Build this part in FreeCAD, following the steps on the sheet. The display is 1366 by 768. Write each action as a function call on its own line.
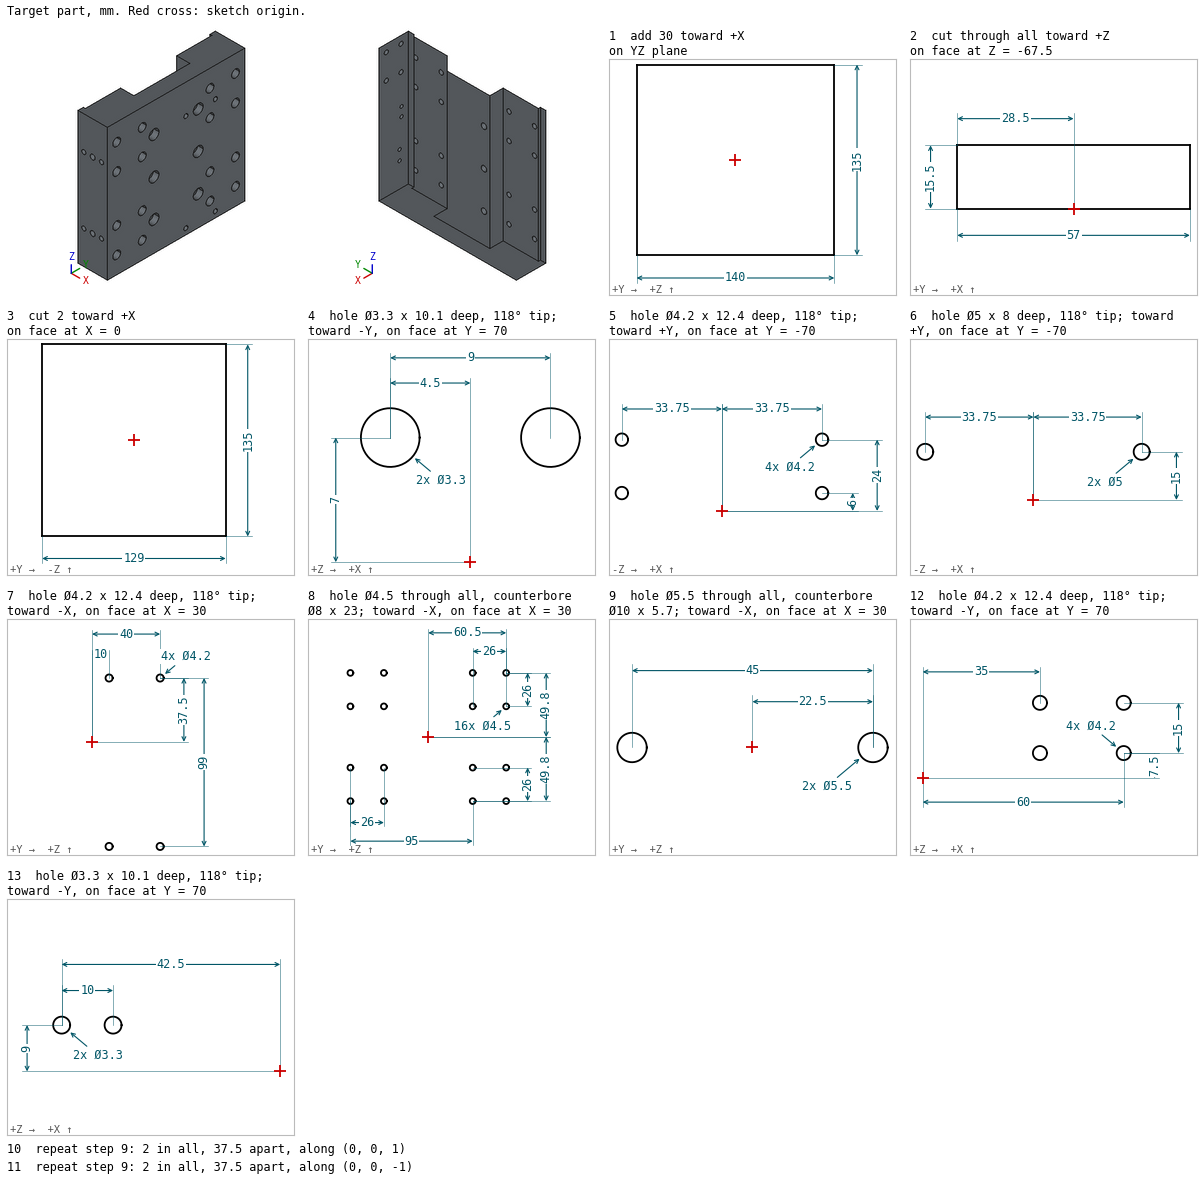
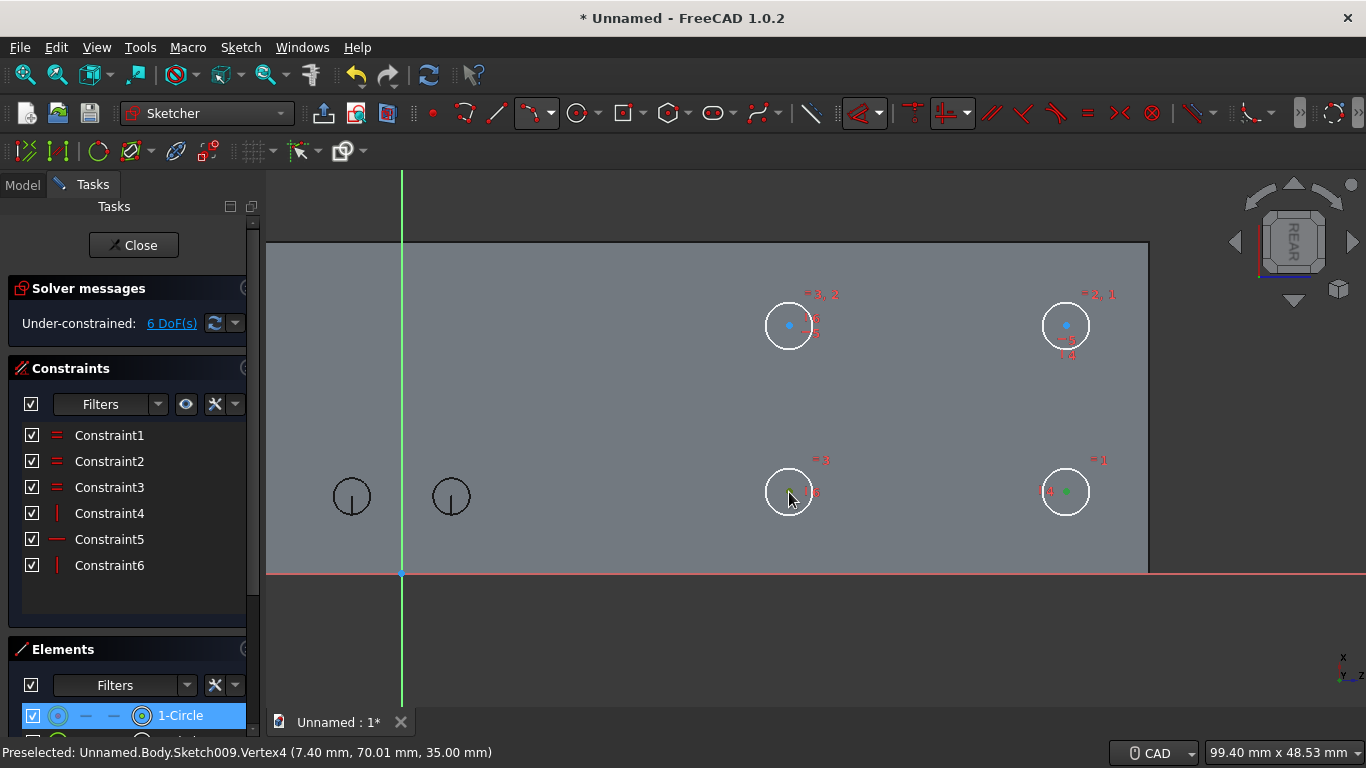
click(970, 114)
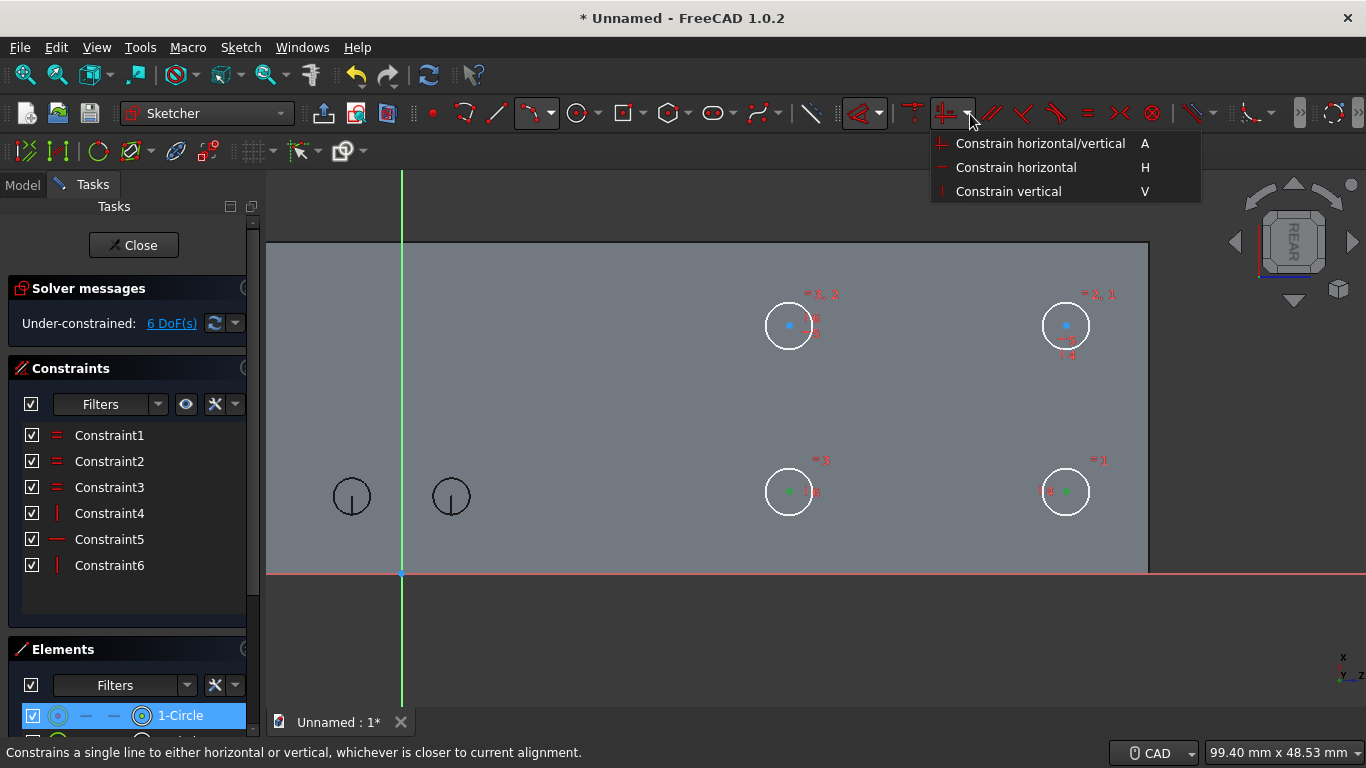
click(1066, 167)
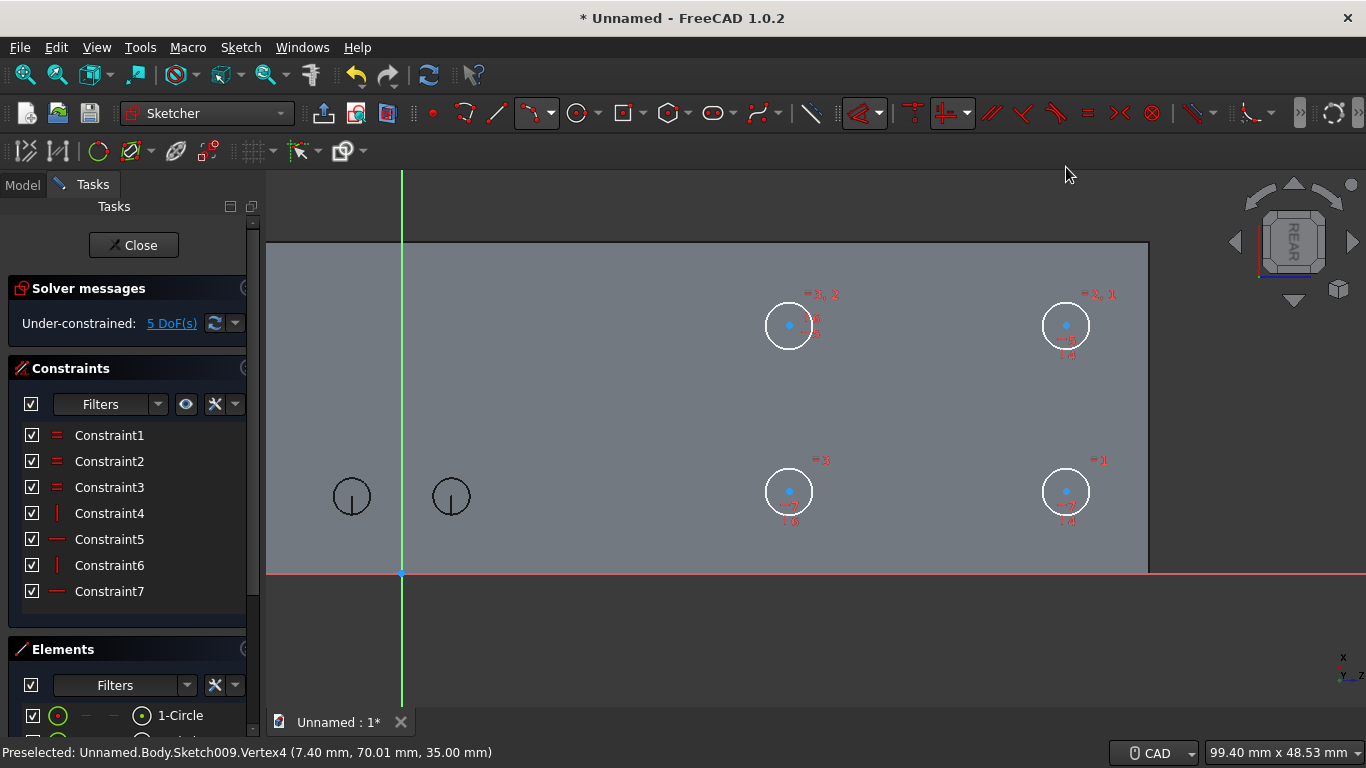
click(1082, 475)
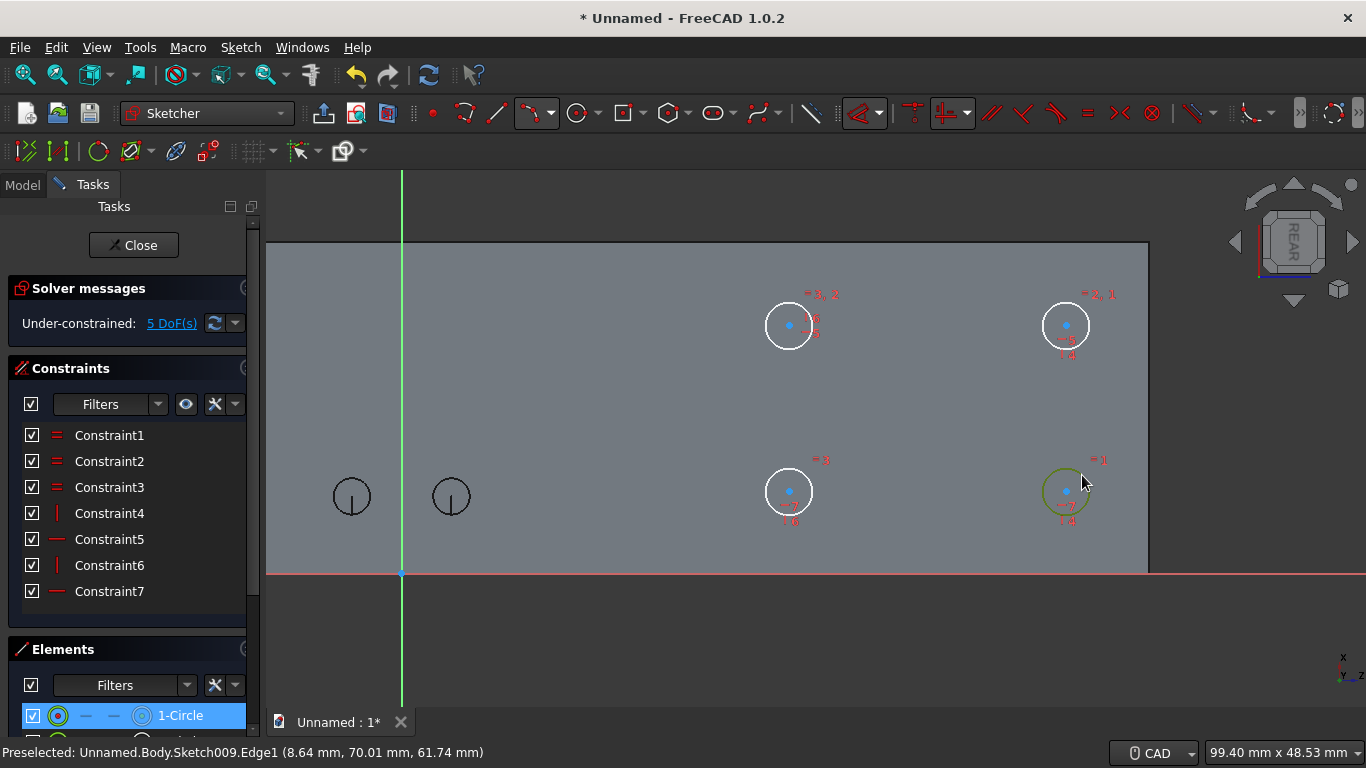
click(882, 114)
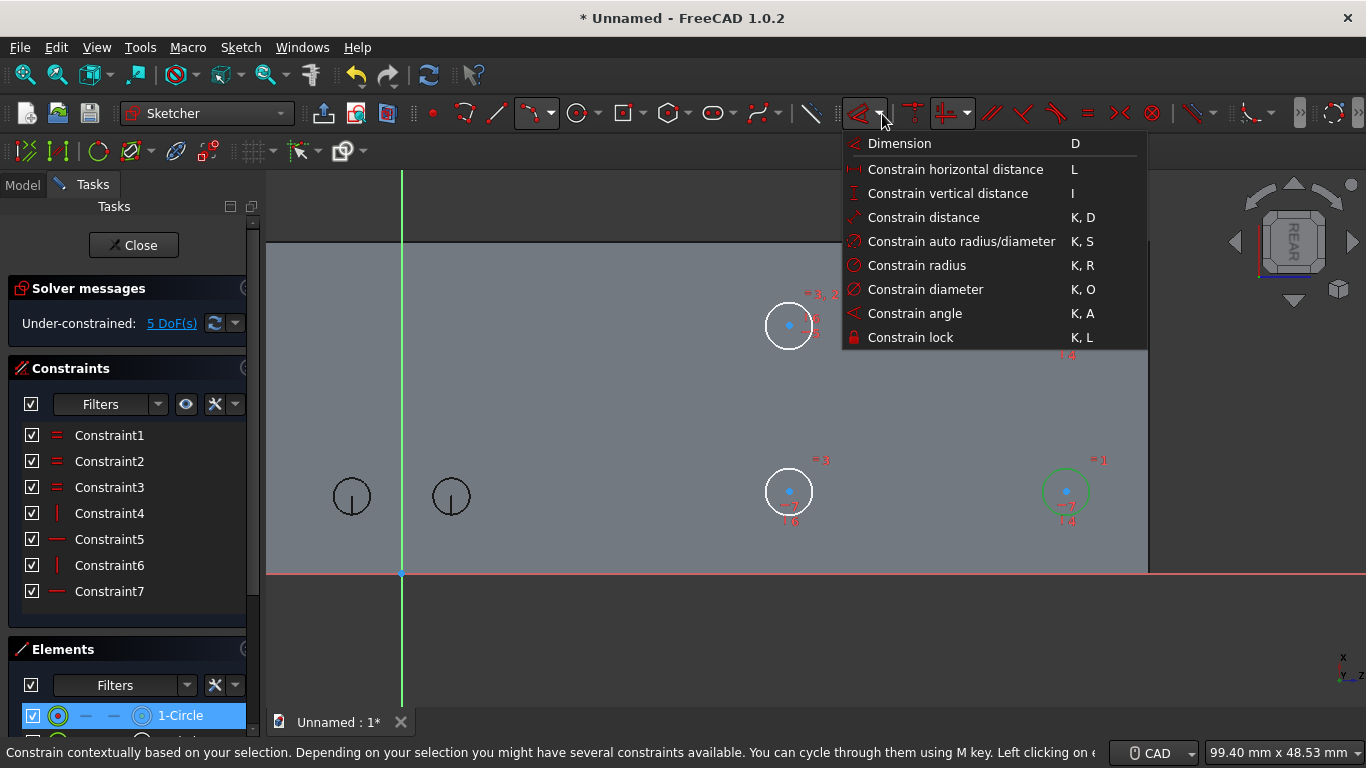
click(995, 289)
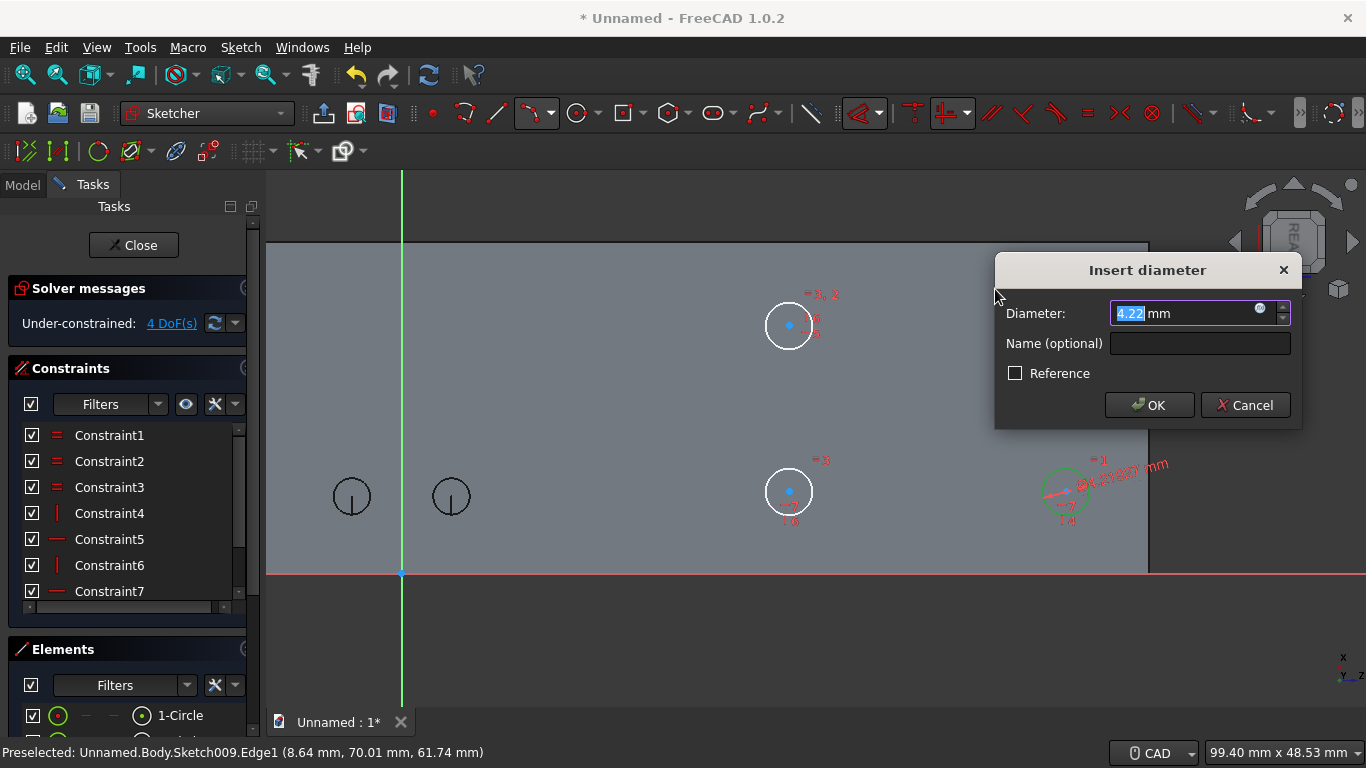
text(4.2)
key(Return)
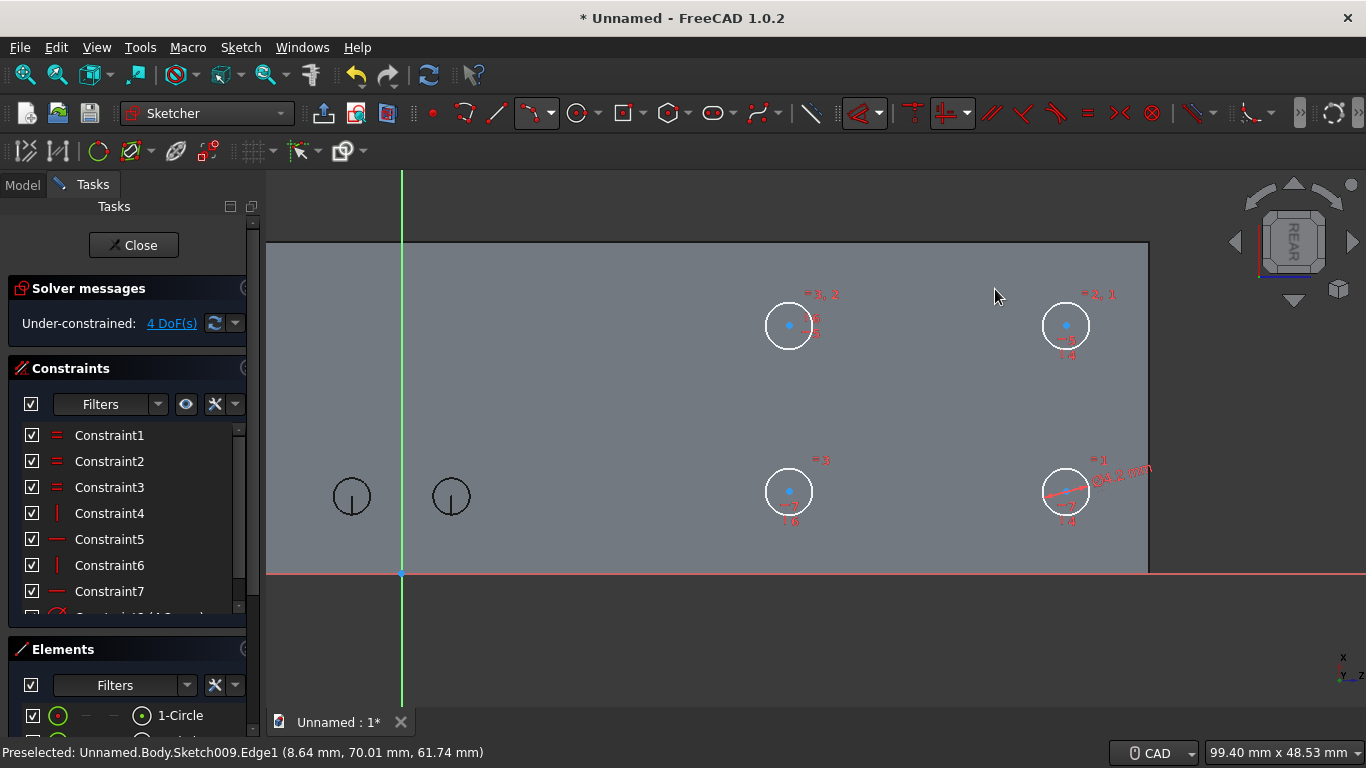
click(1066, 492)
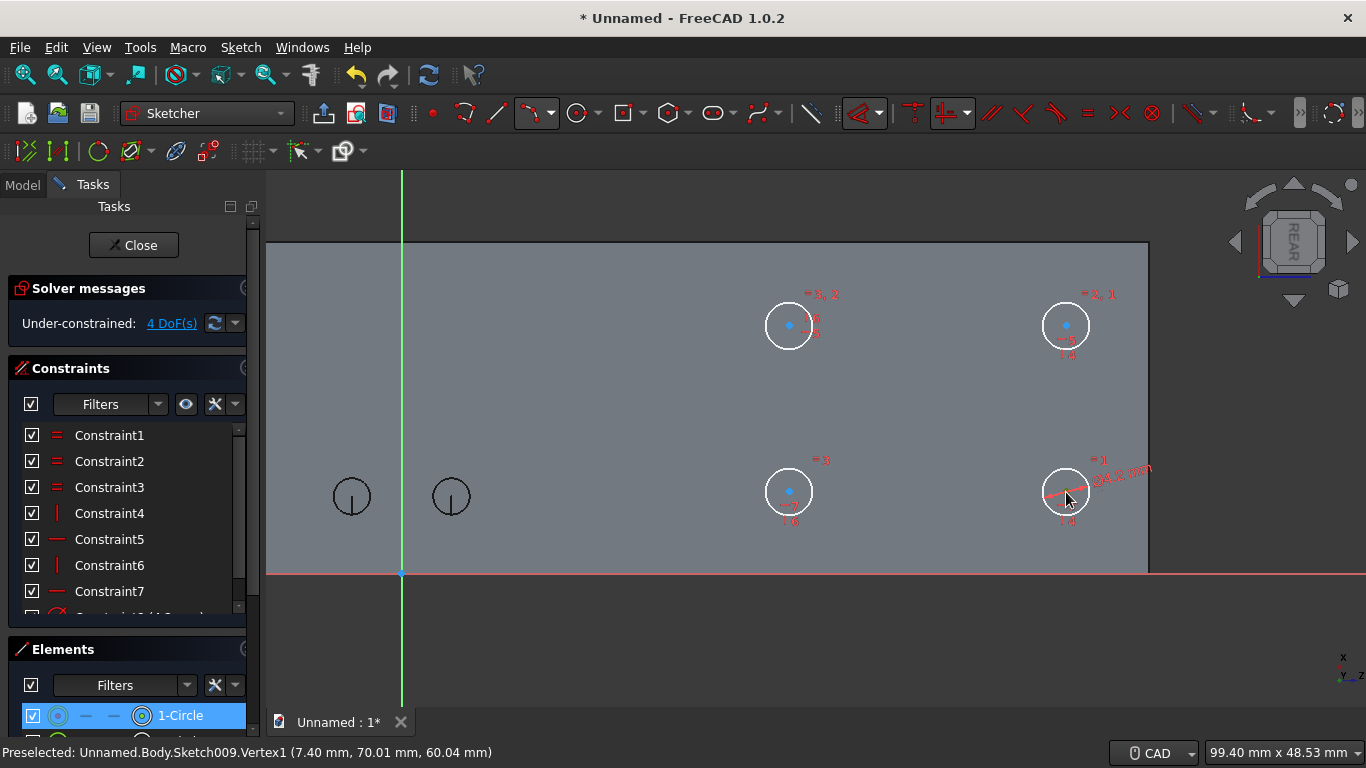
click(882, 114)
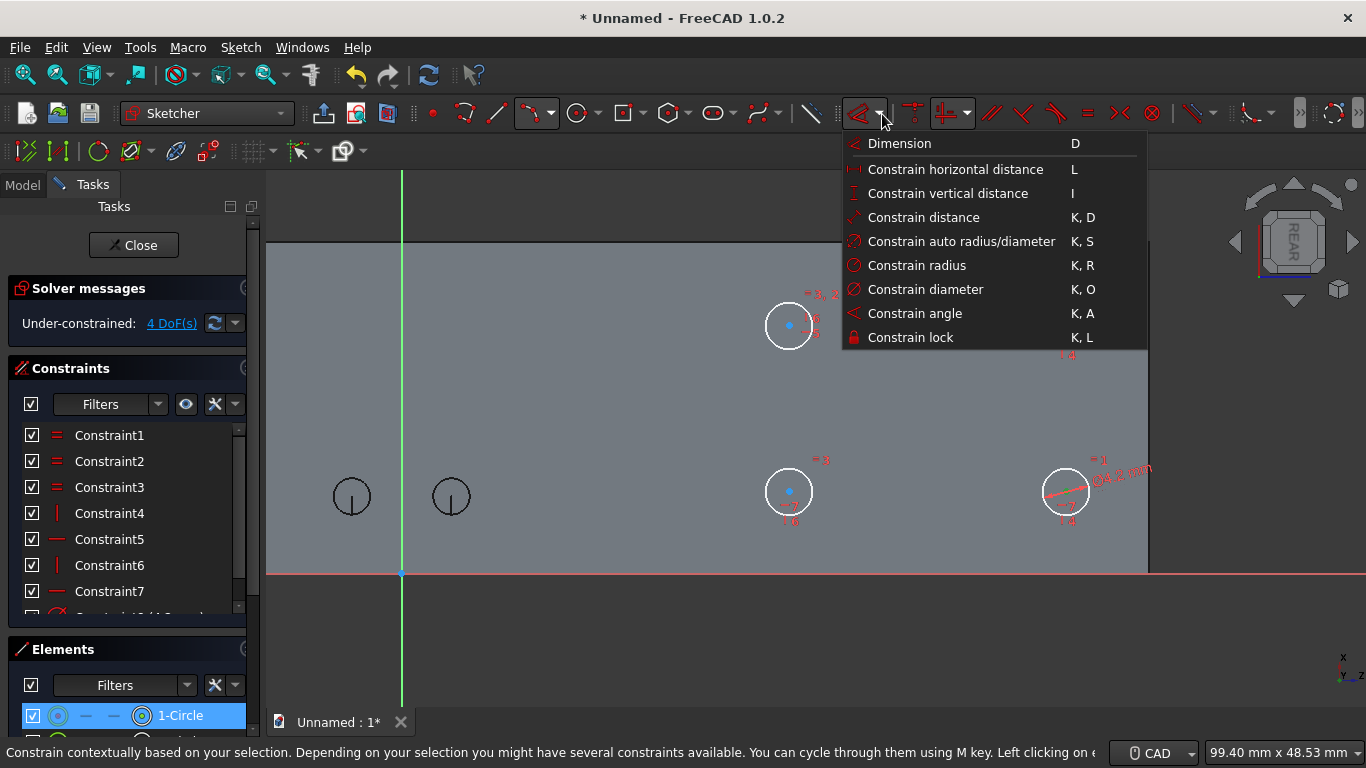
click(995, 169)